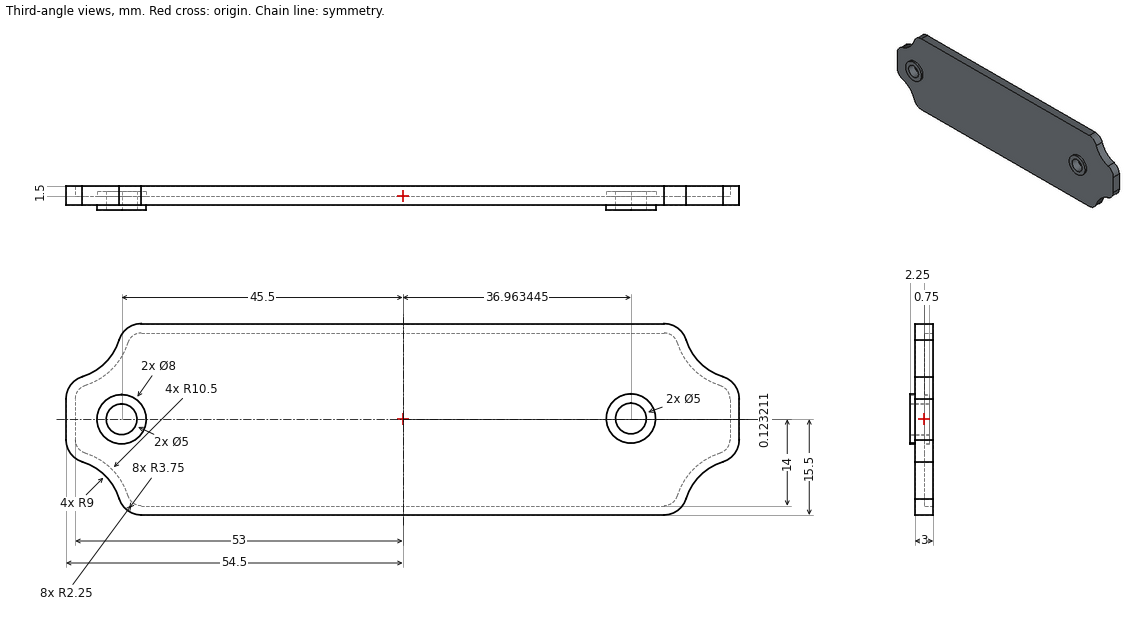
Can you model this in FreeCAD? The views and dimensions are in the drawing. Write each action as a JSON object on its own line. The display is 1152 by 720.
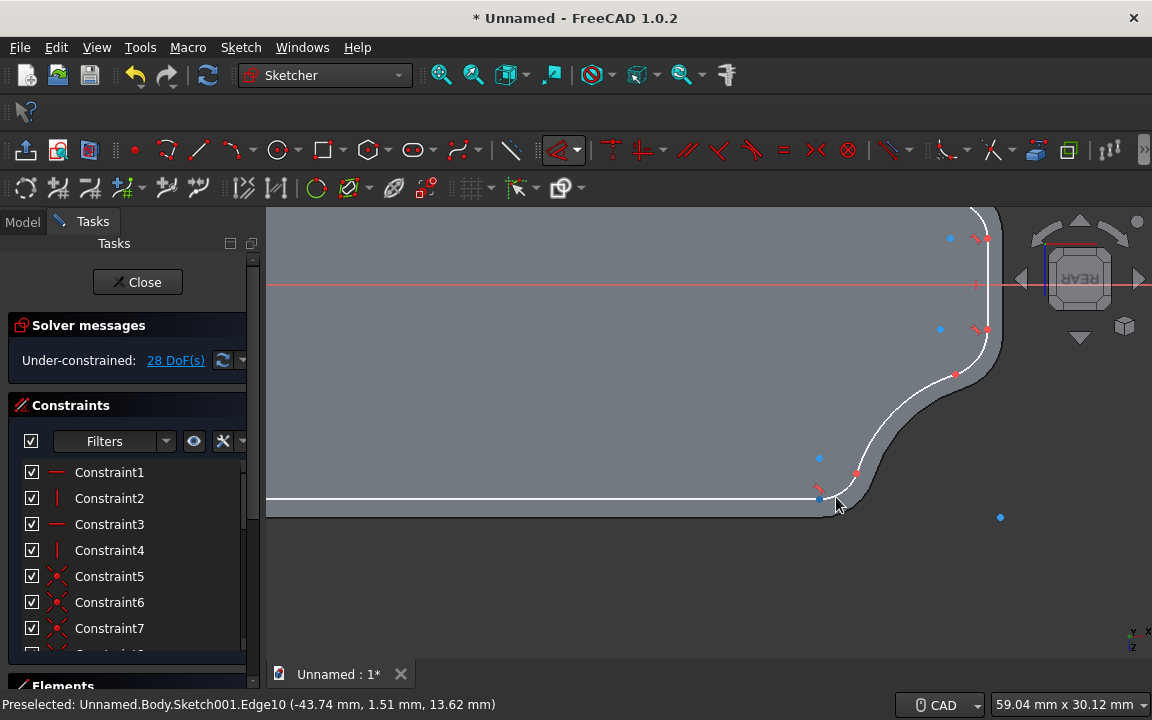
{"action": "left_click", "coordinate": [834, 497]}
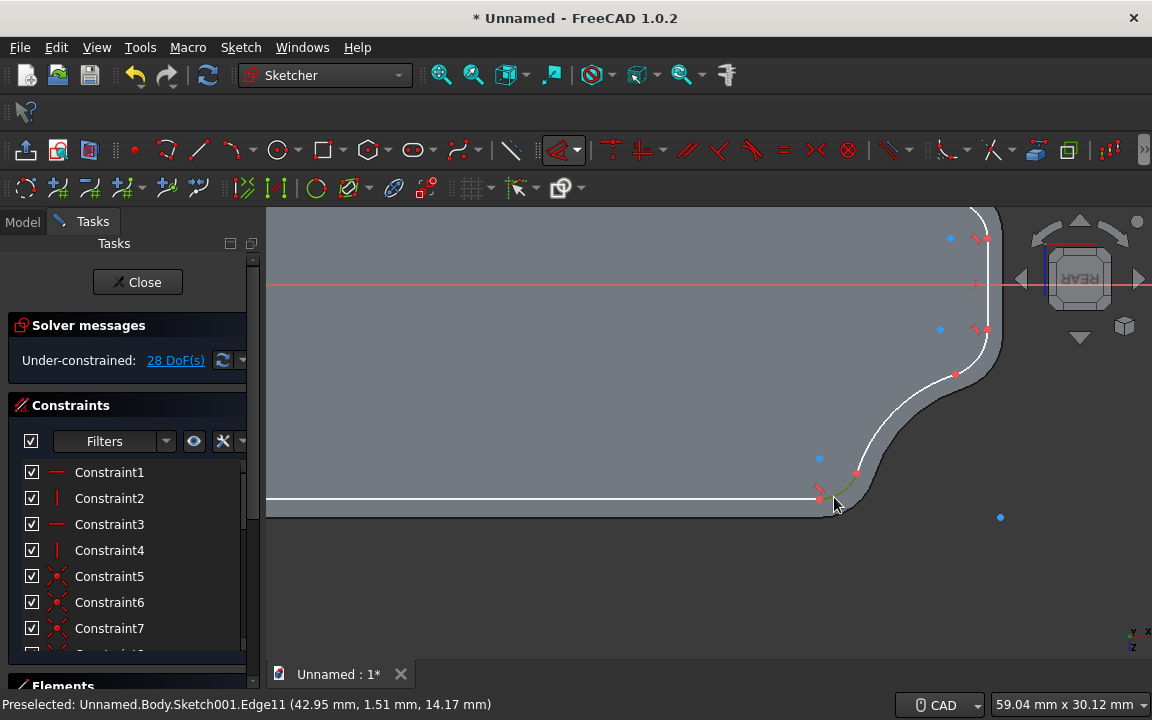
{"action": "left_click", "coordinate": [917, 393]}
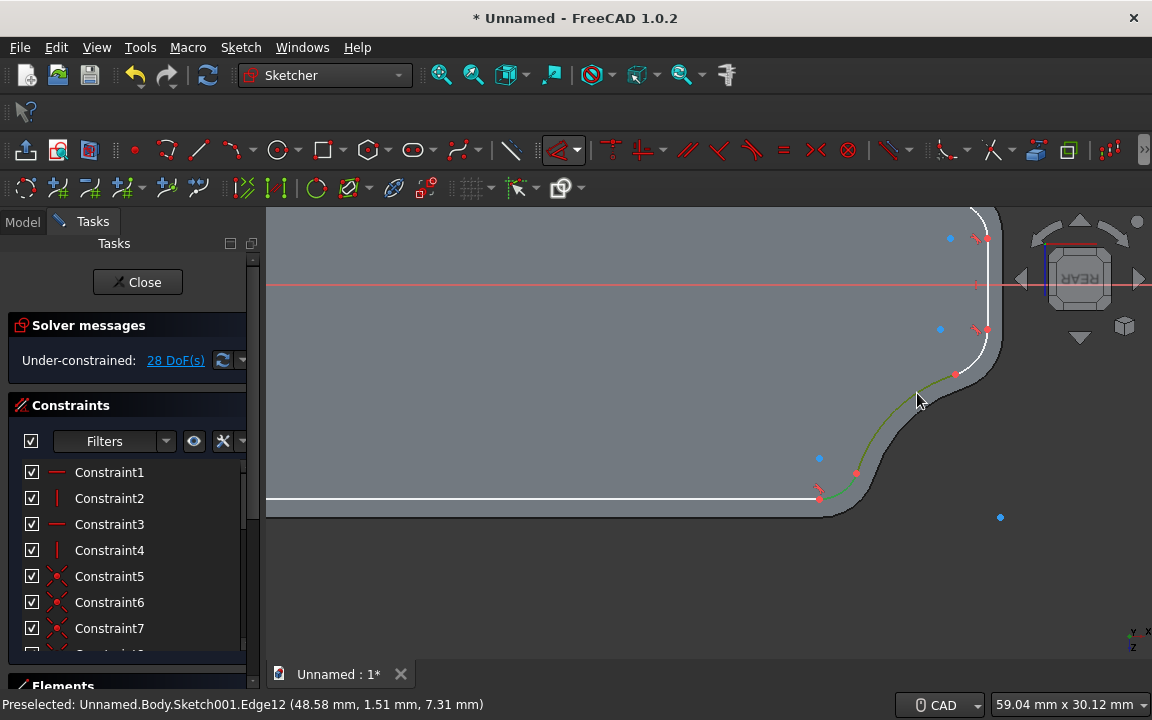
{"action": "left_click", "coordinate": [752, 150]}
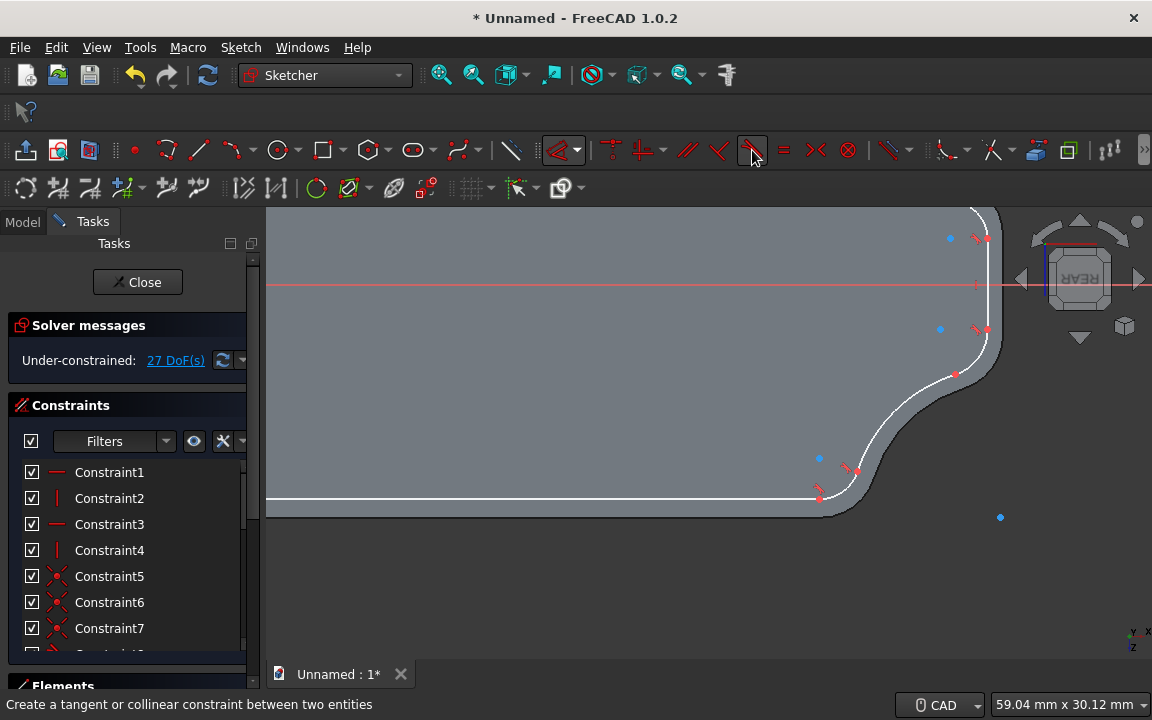
{"action": "left_click", "coordinate": [917, 393]}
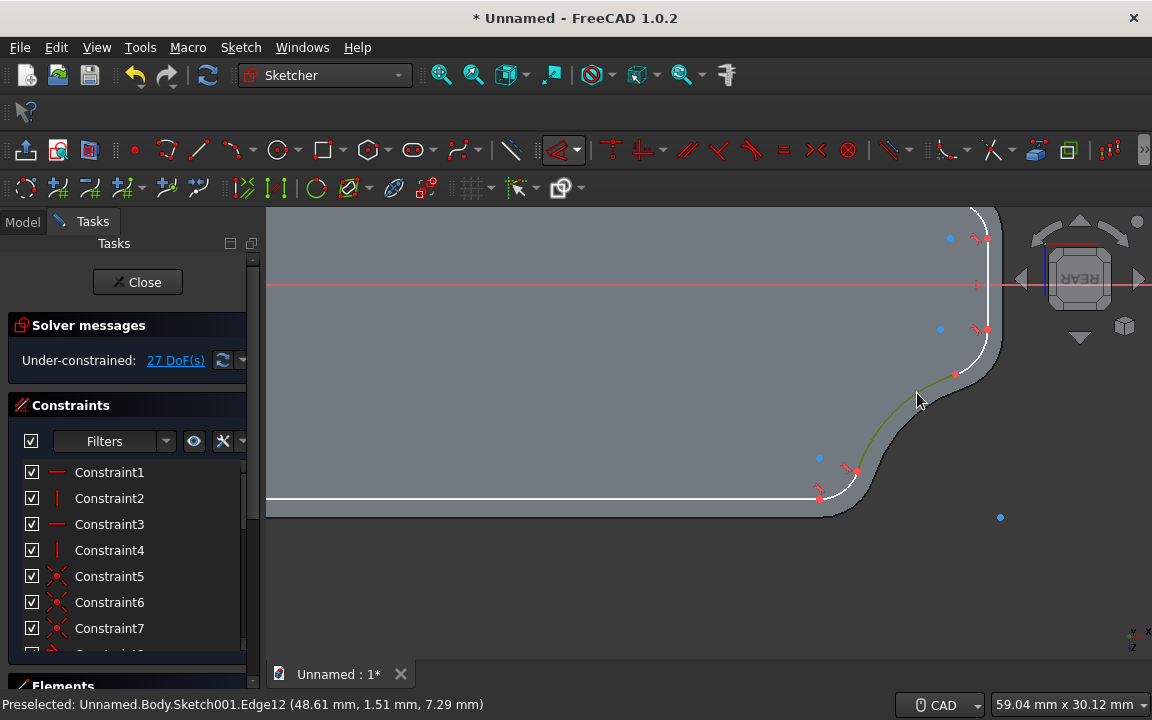
{"action": "left_click", "coordinate": [971, 366]}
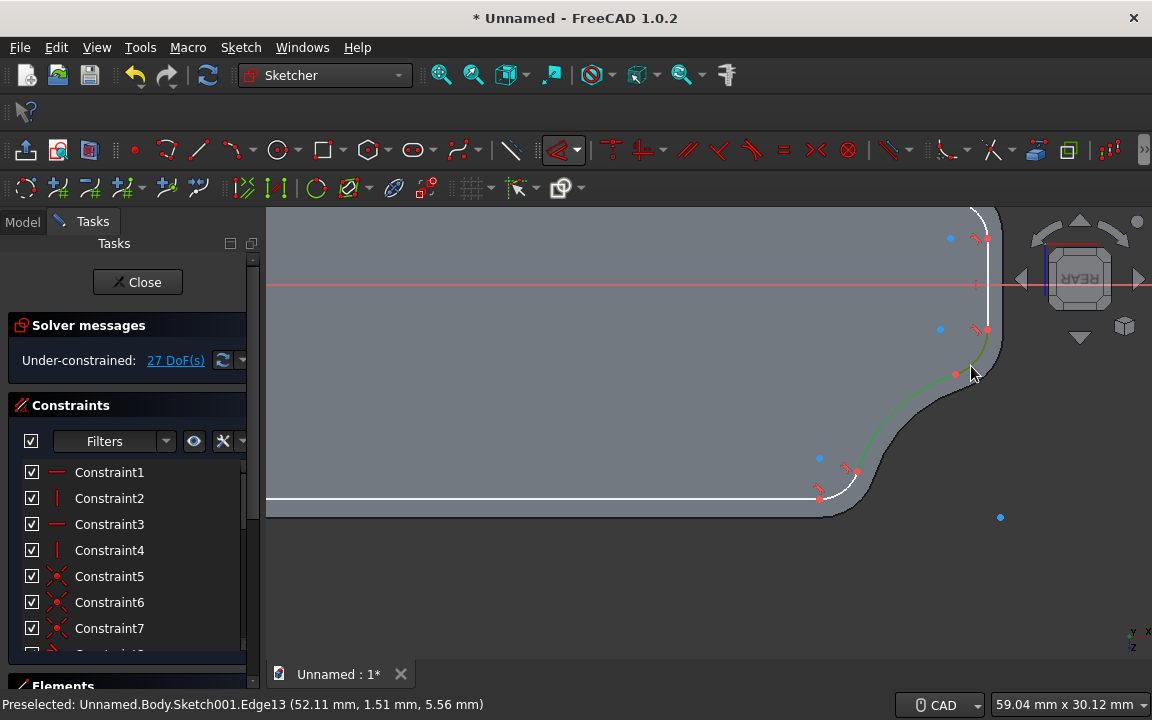
{"action": "left_click", "coordinate": [752, 150]}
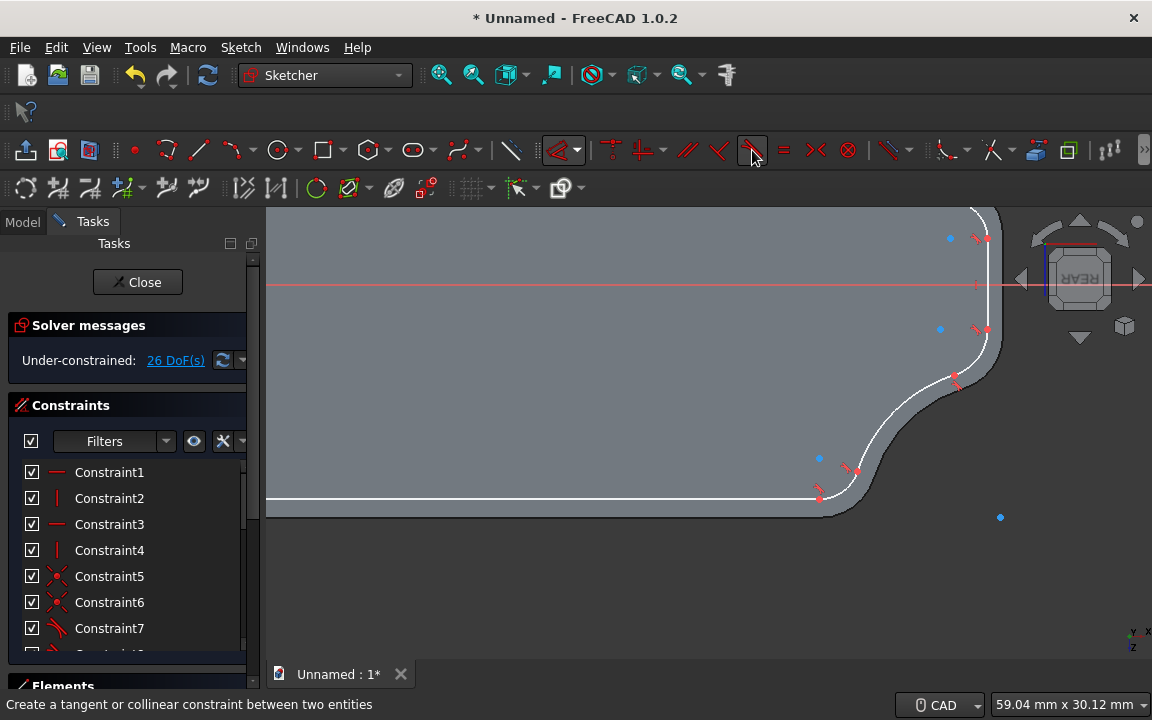
{"action": "scroll", "coordinate": [837, 497], "scroll_direction": "down", "scroll_amount": 6}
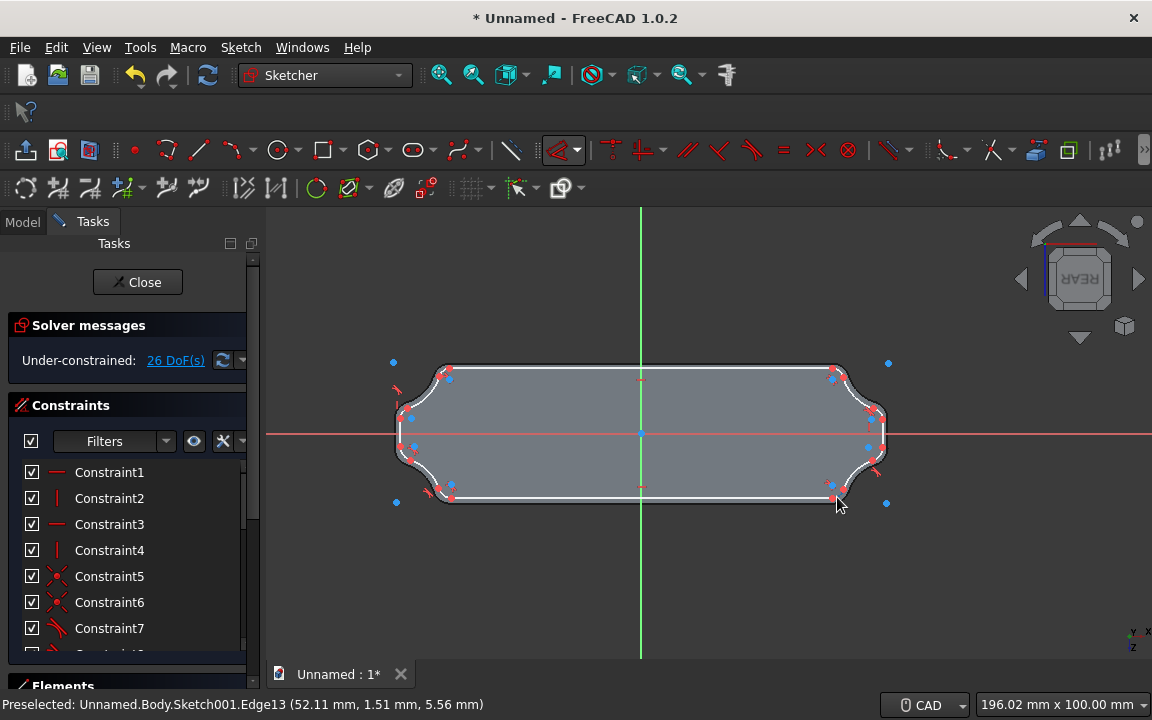
{"action": "scroll", "coordinate": [882, 415], "scroll_direction": "up", "scroll_amount": 6}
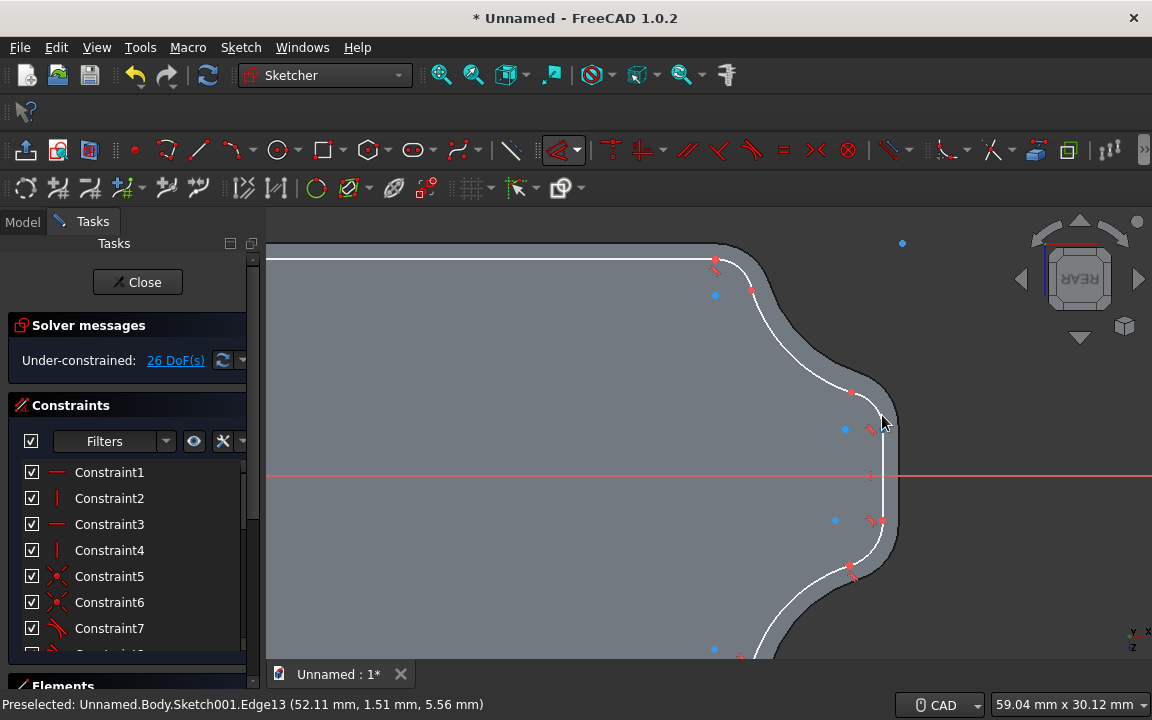
{"action": "left_click", "coordinate": [880, 414]}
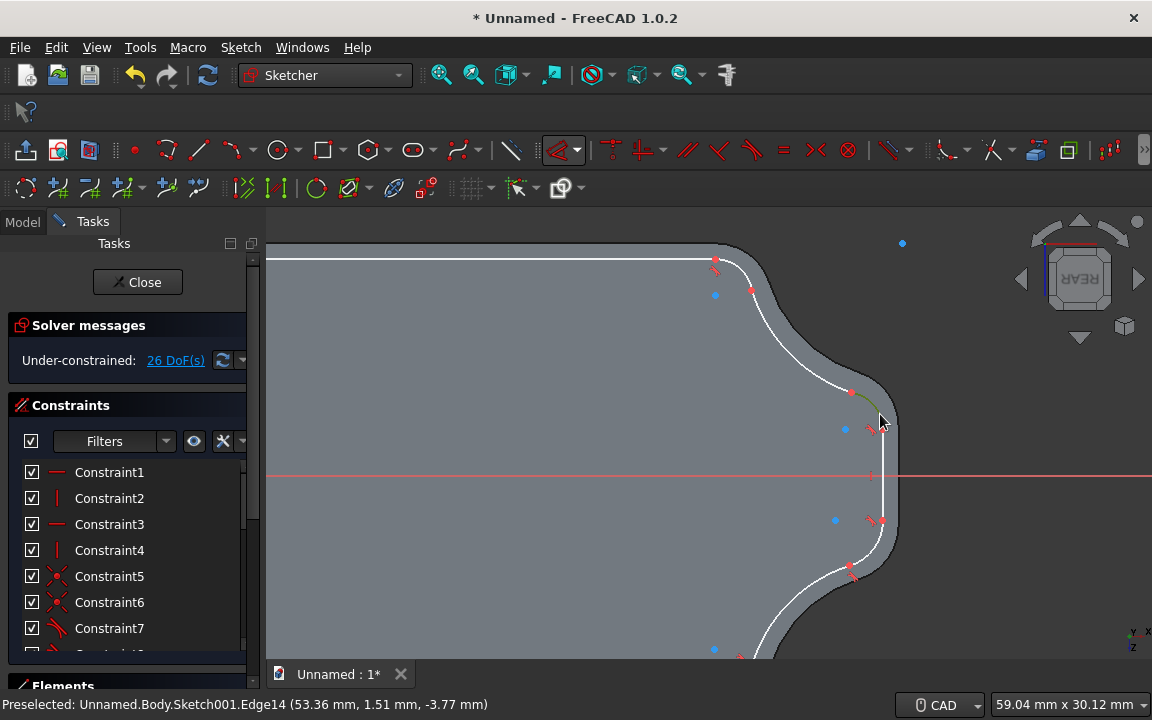
{"action": "left_click", "coordinate": [771, 331]}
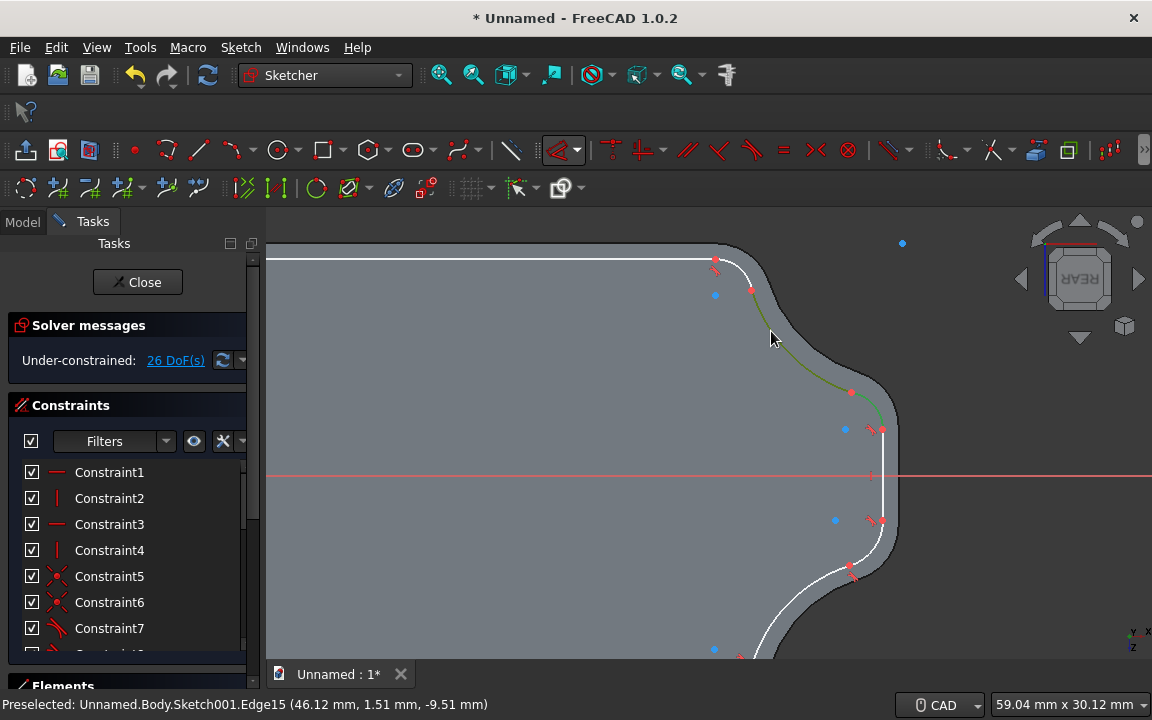
{"action": "left_click", "coordinate": [752, 150]}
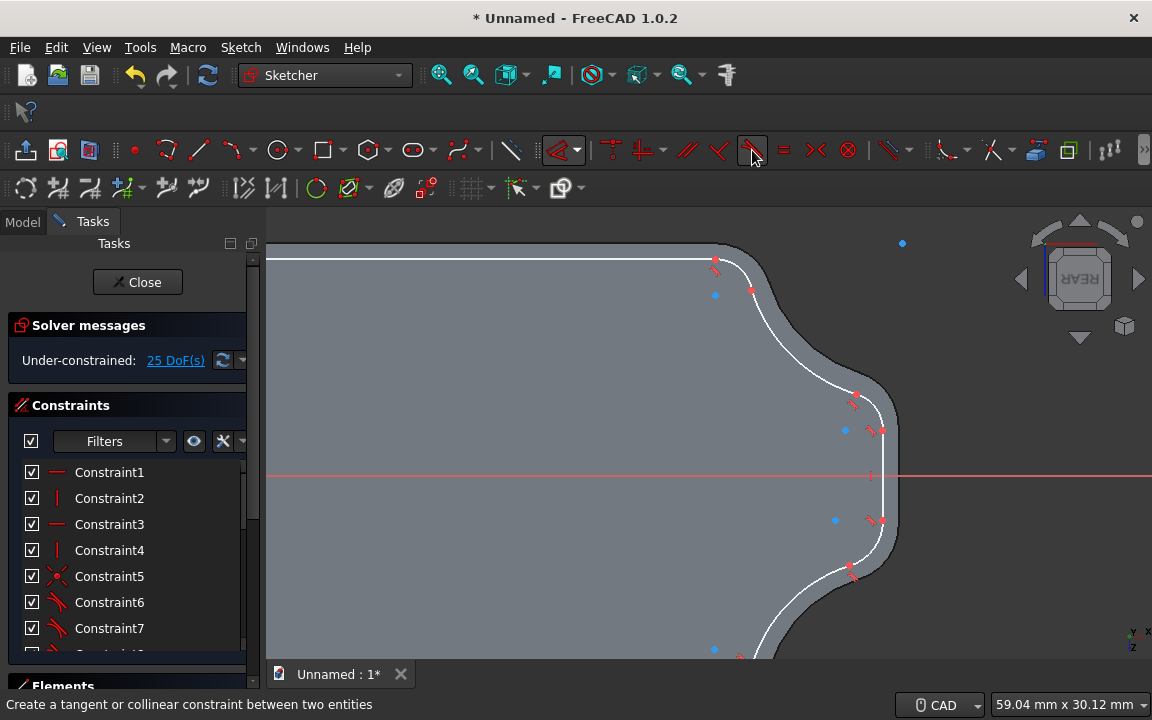
{"action": "left_click", "coordinate": [772, 332]}